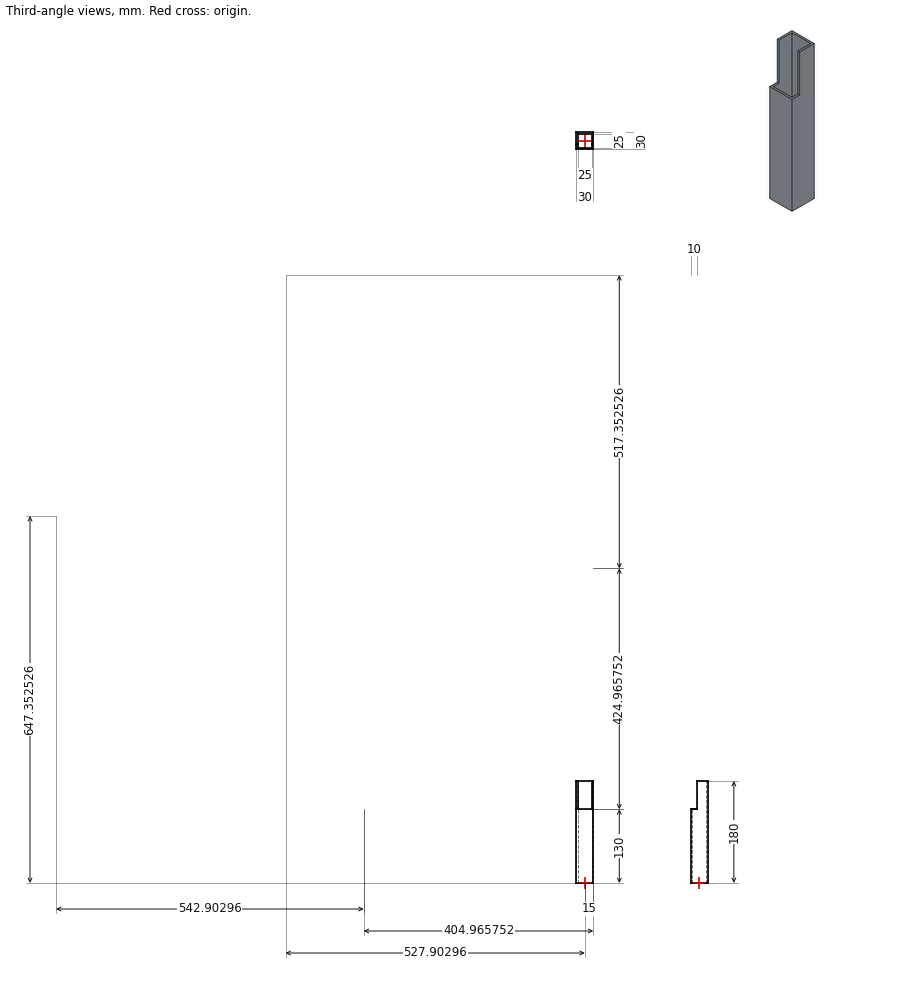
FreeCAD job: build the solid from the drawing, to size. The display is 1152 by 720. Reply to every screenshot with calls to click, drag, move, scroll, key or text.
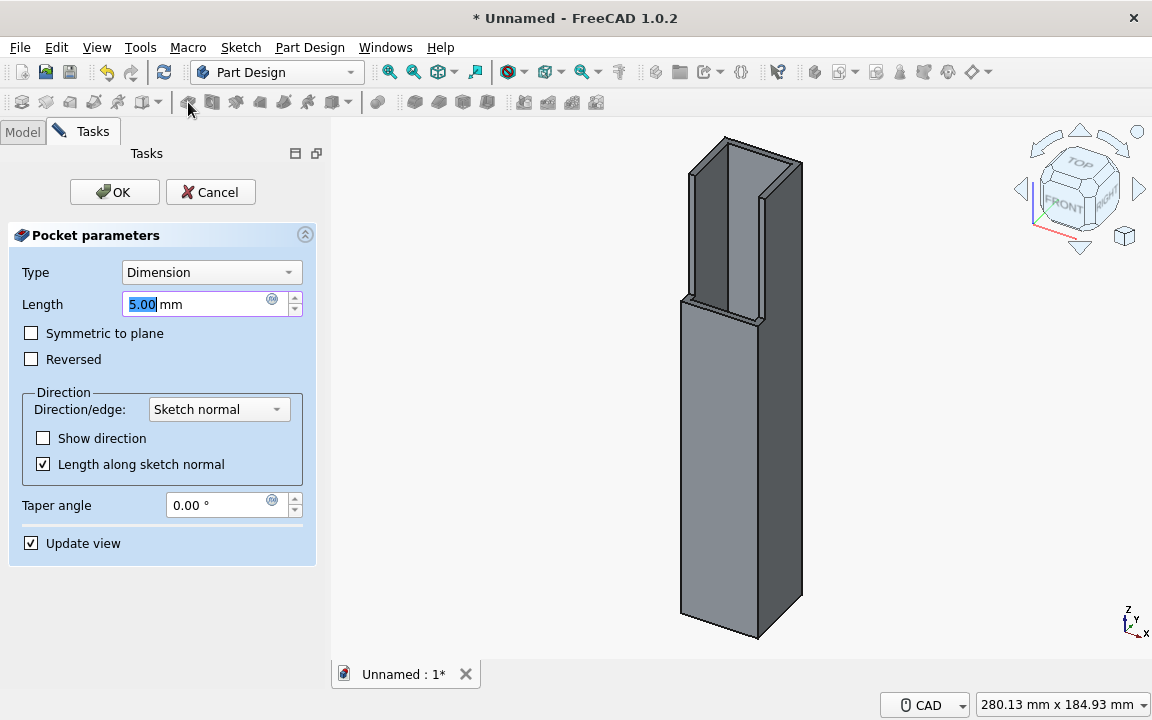
click(212, 272)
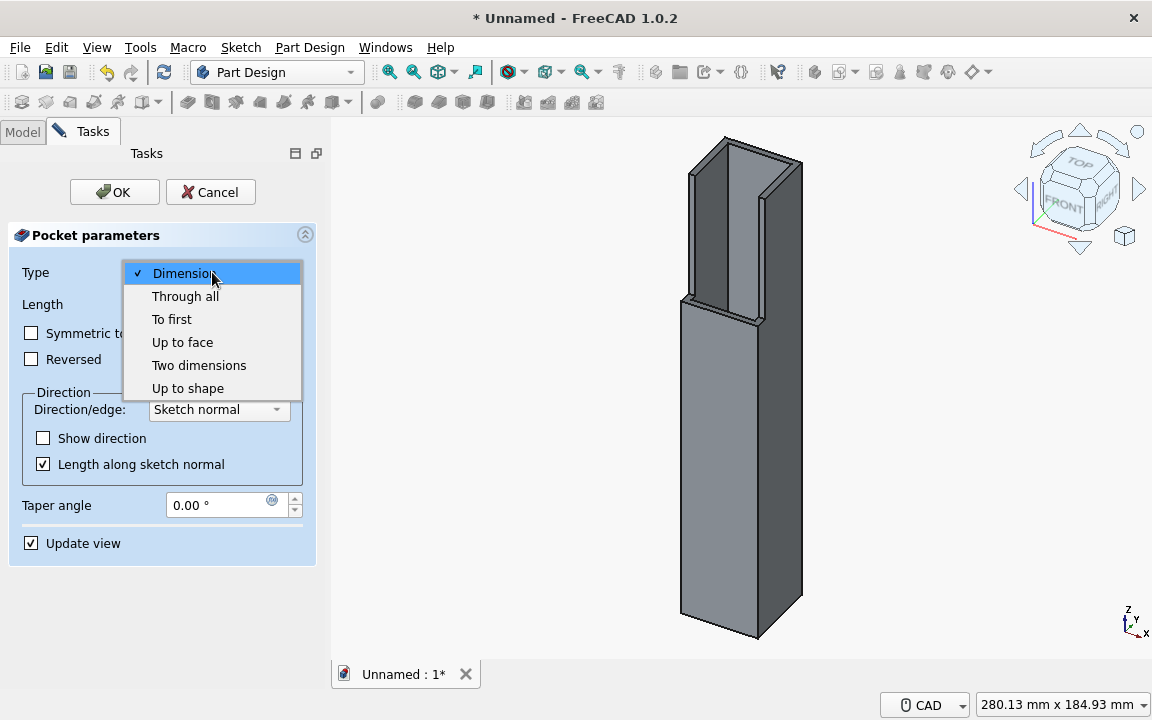
click(212, 366)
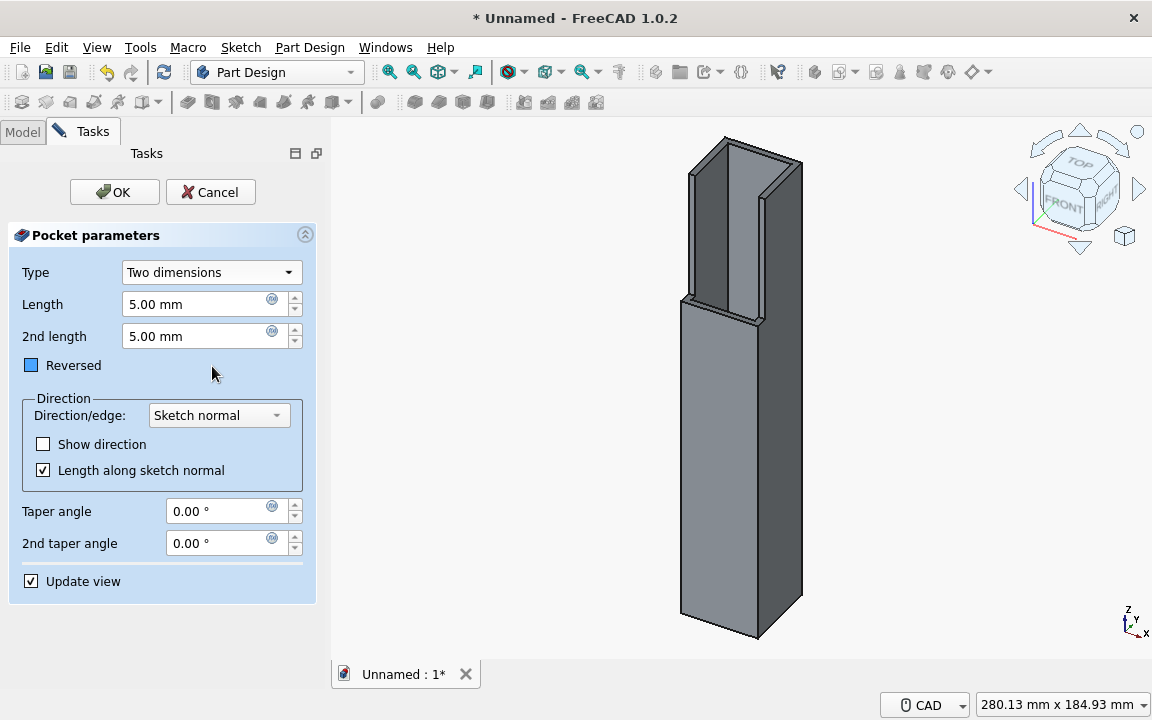
triple_click(204, 304)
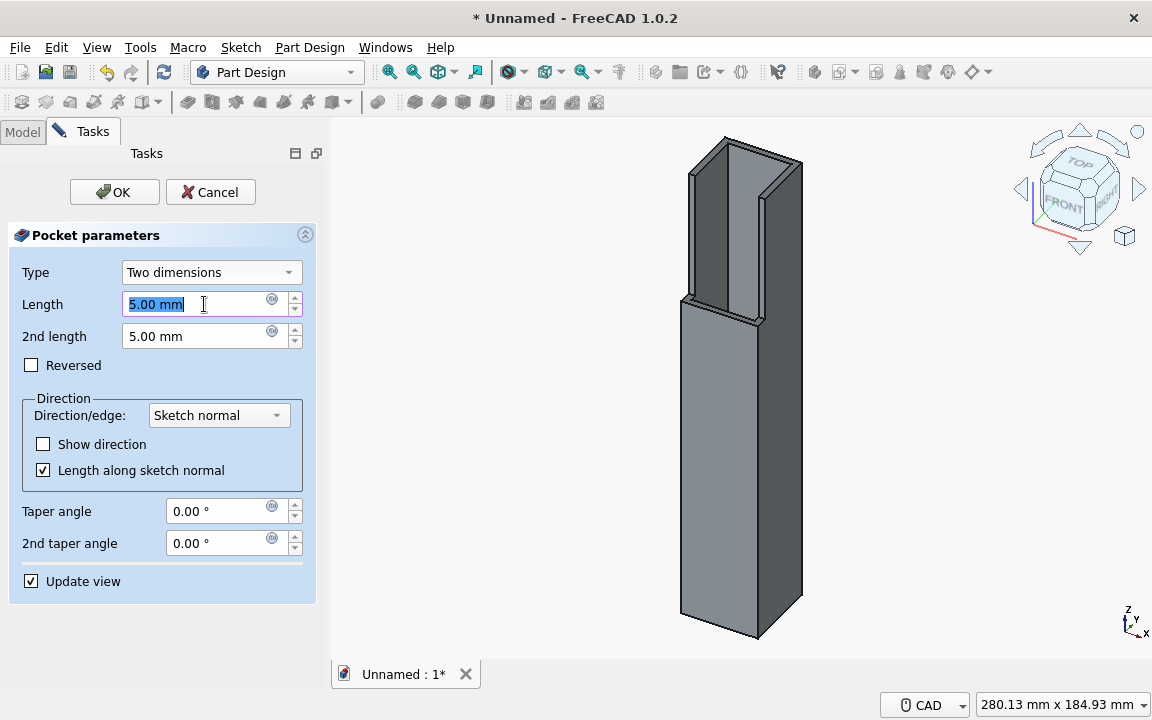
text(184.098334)
key(Tab)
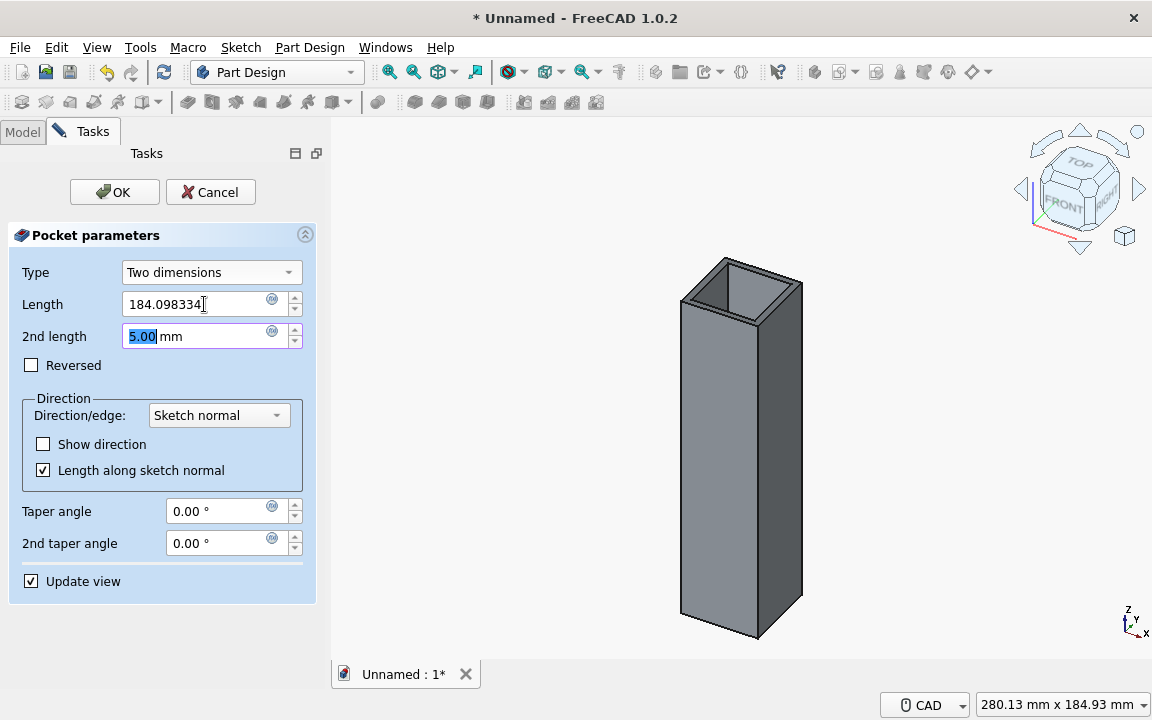
text(10)
key(Tab)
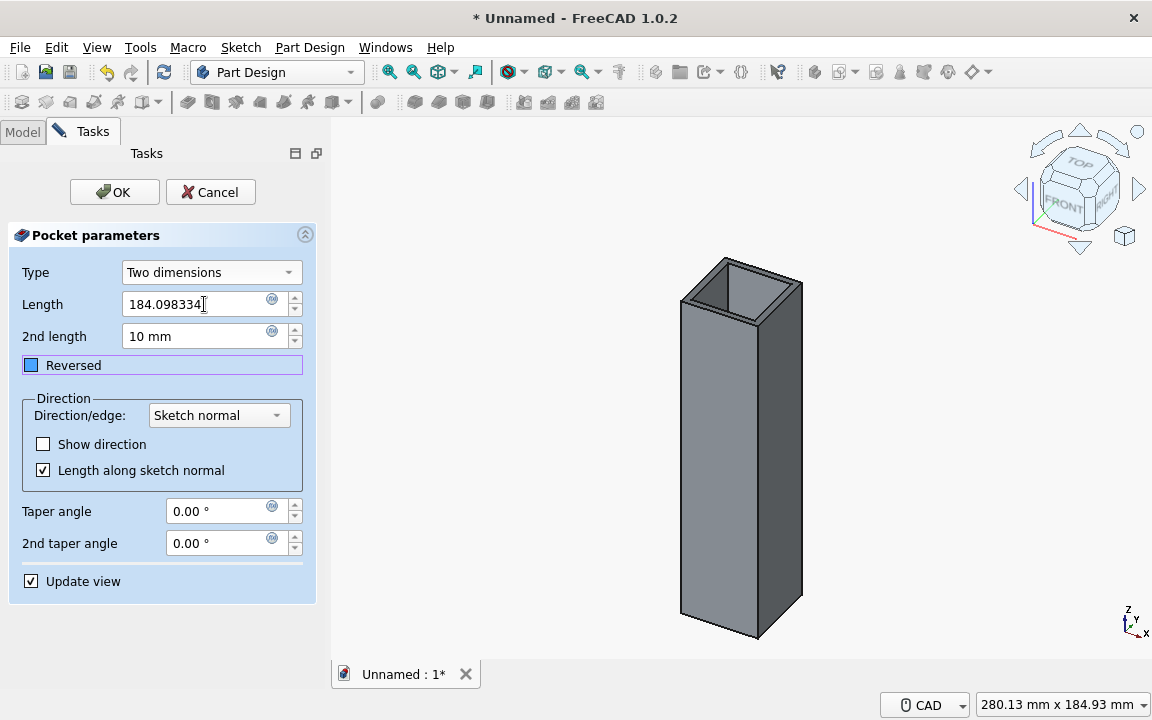
click(30, 365)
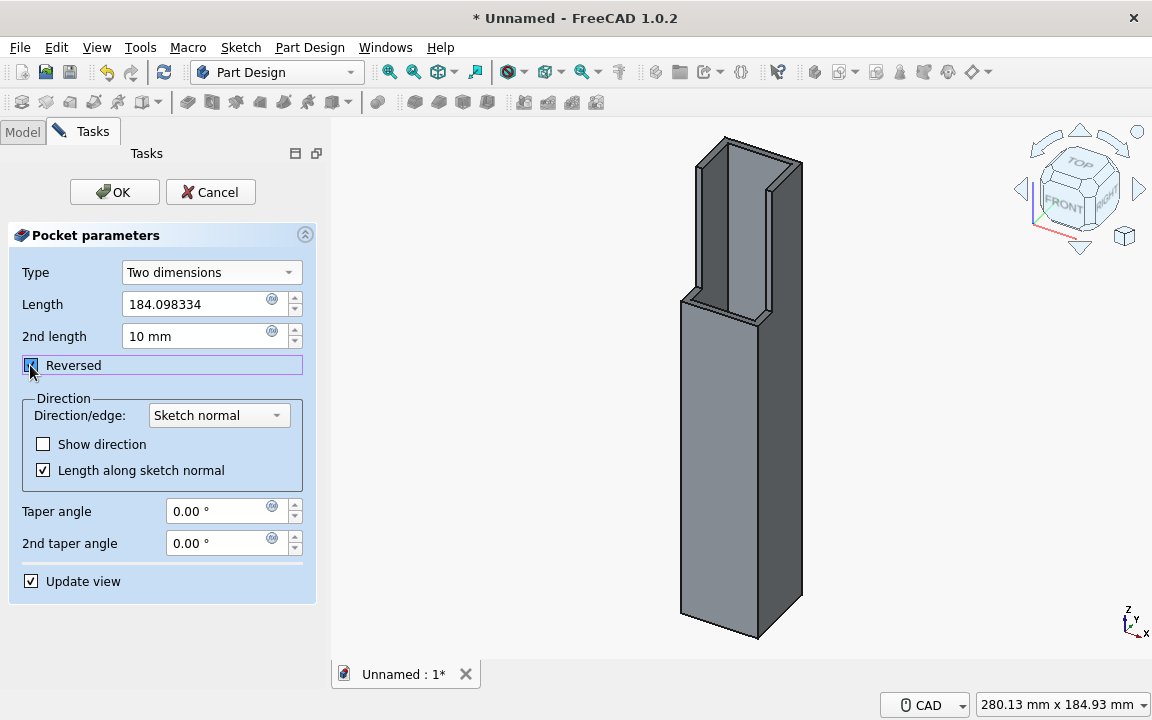
click(115, 192)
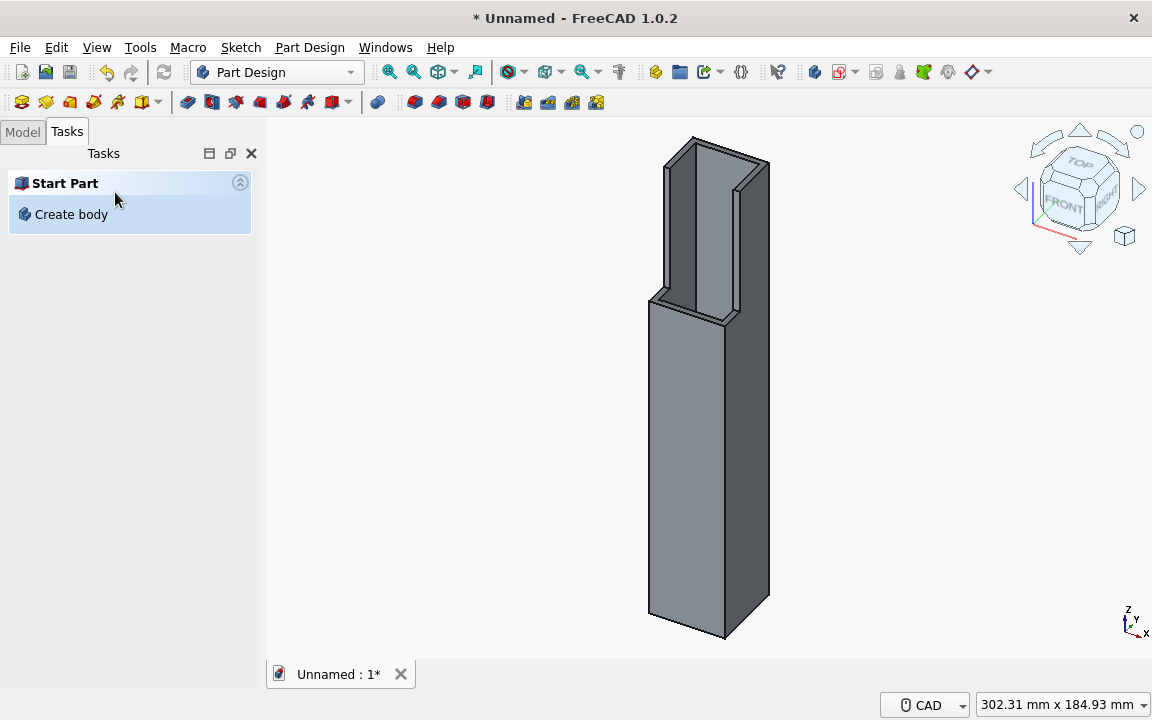
key(0)